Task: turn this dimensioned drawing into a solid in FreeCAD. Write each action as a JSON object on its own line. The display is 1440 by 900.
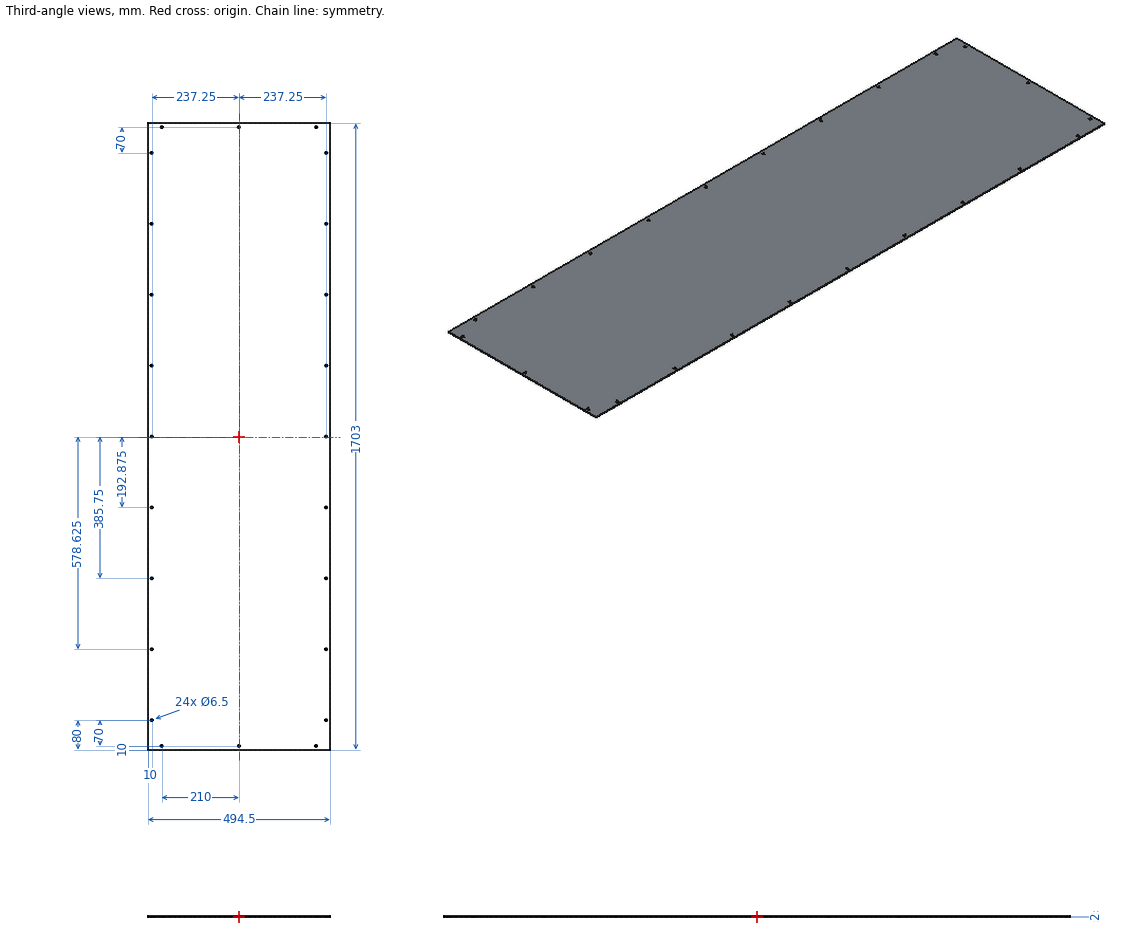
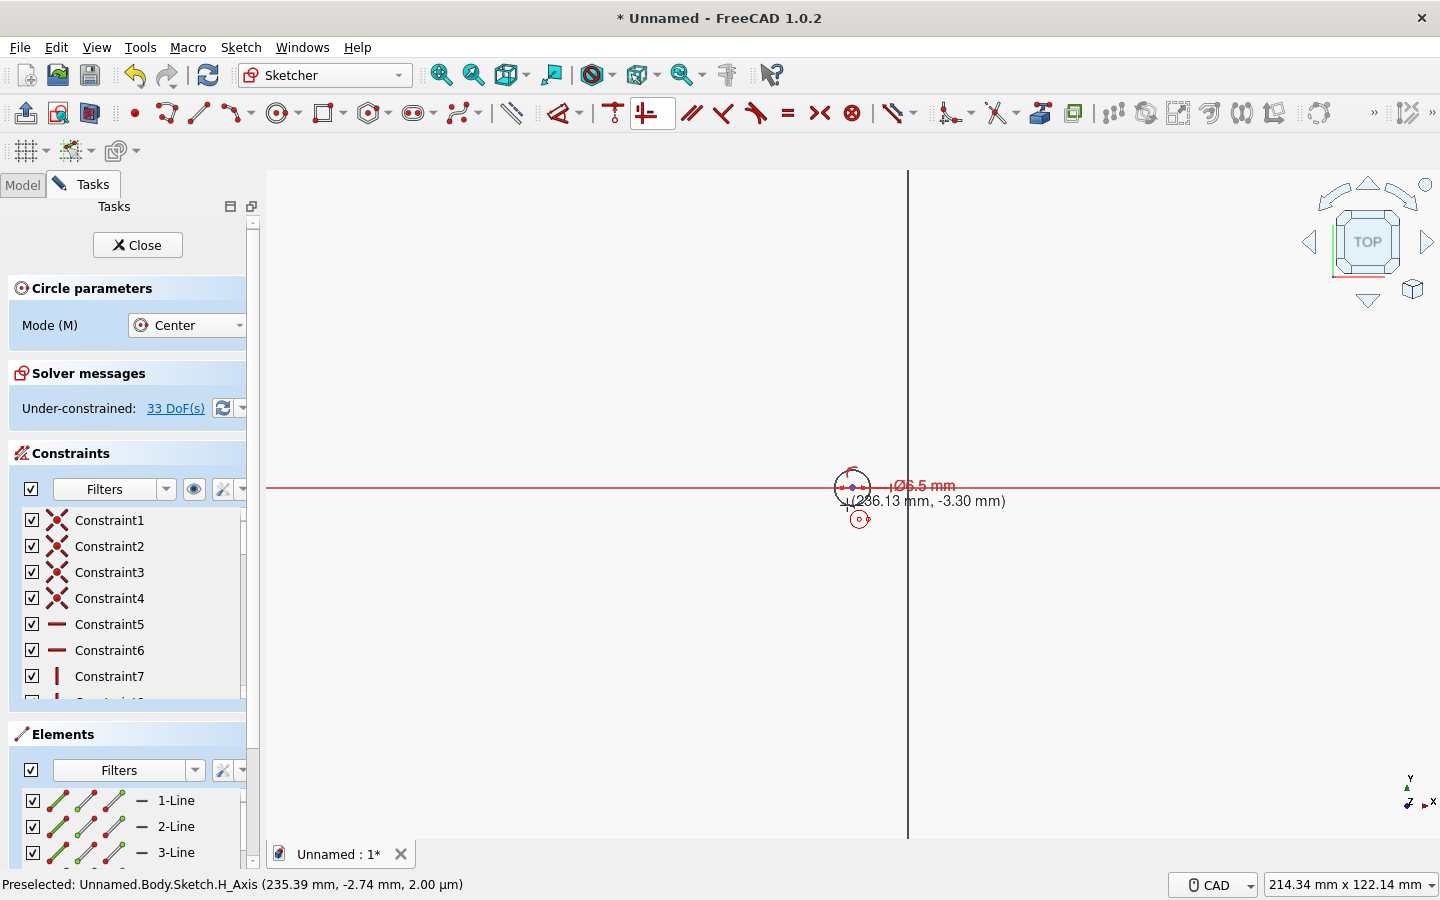
{"action": "scroll", "coordinate": [849, 505], "scroll_direction": "down", "scroll_amount": 15}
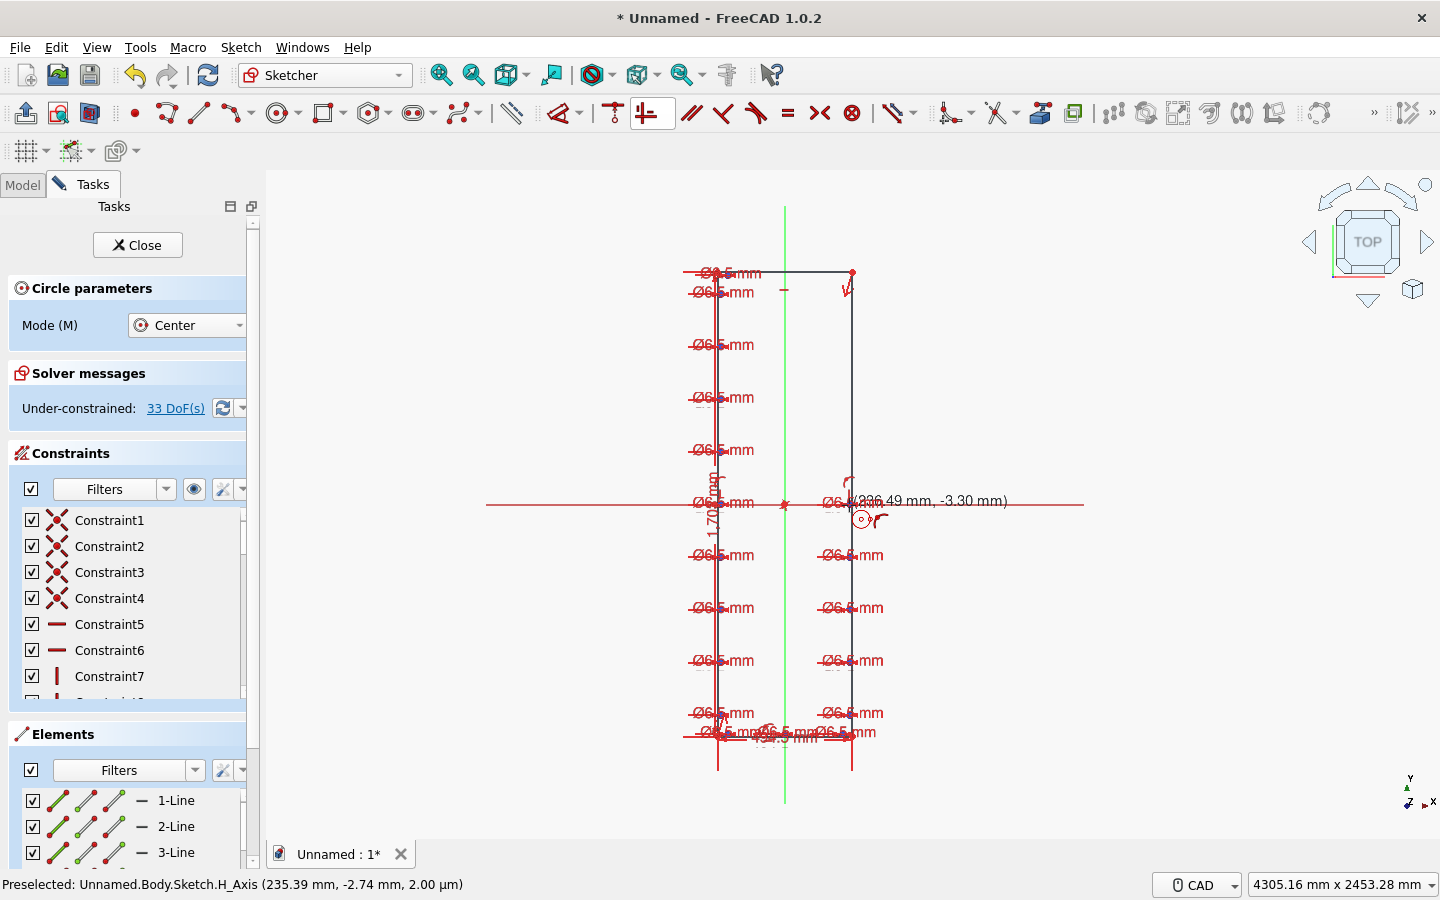
{"action": "scroll", "coordinate": [850, 452], "scroll_direction": "up", "scroll_amount": 17}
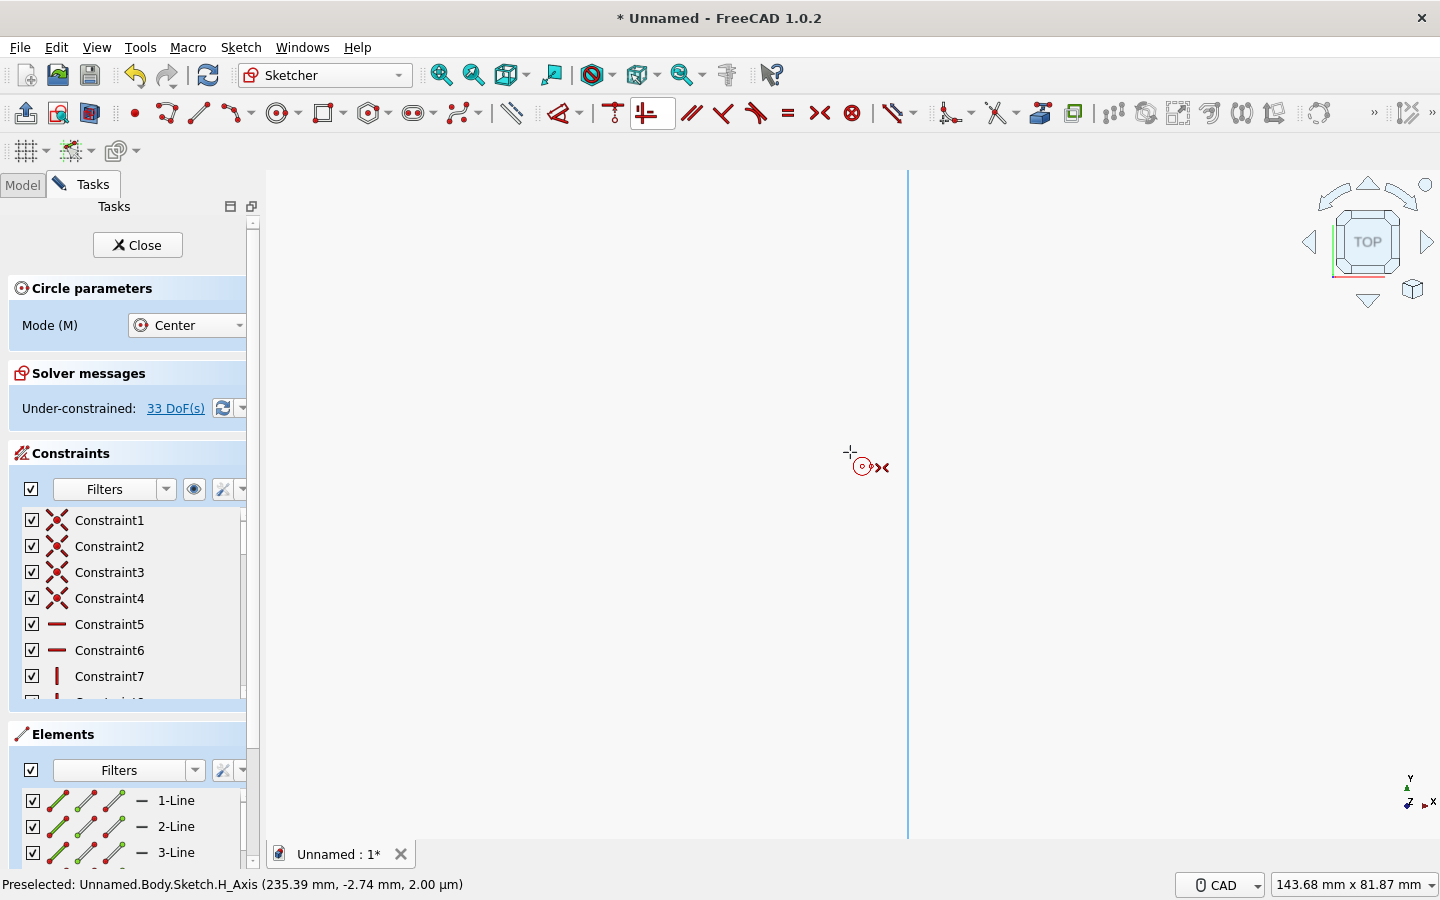
{"action": "scroll", "coordinate": [850, 452], "scroll_direction": "down", "scroll_amount": 17}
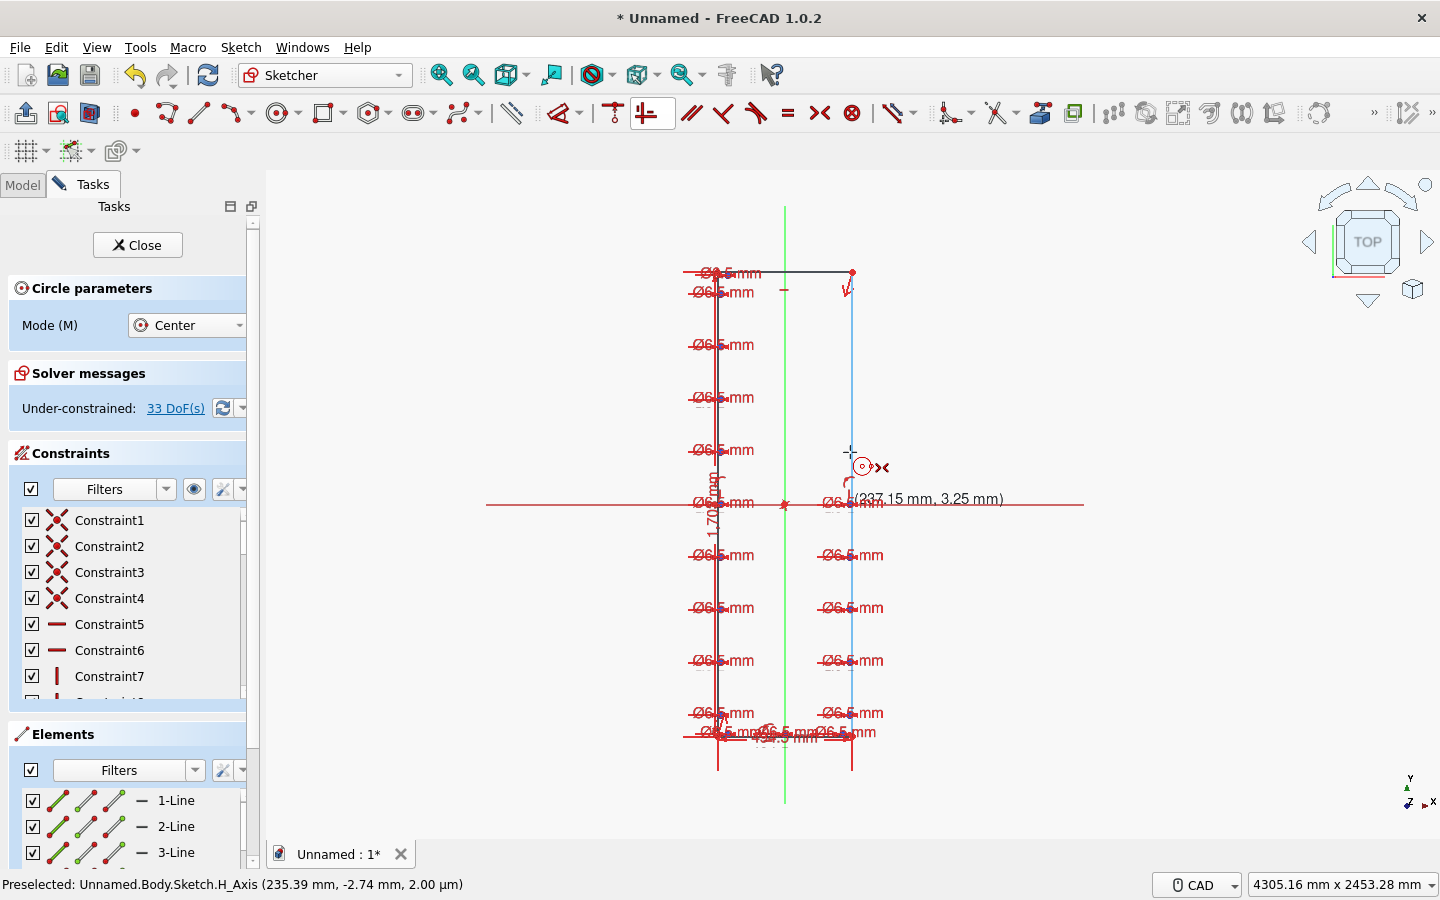
{"action": "scroll", "coordinate": [850, 452], "scroll_direction": "up", "scroll_amount": 9}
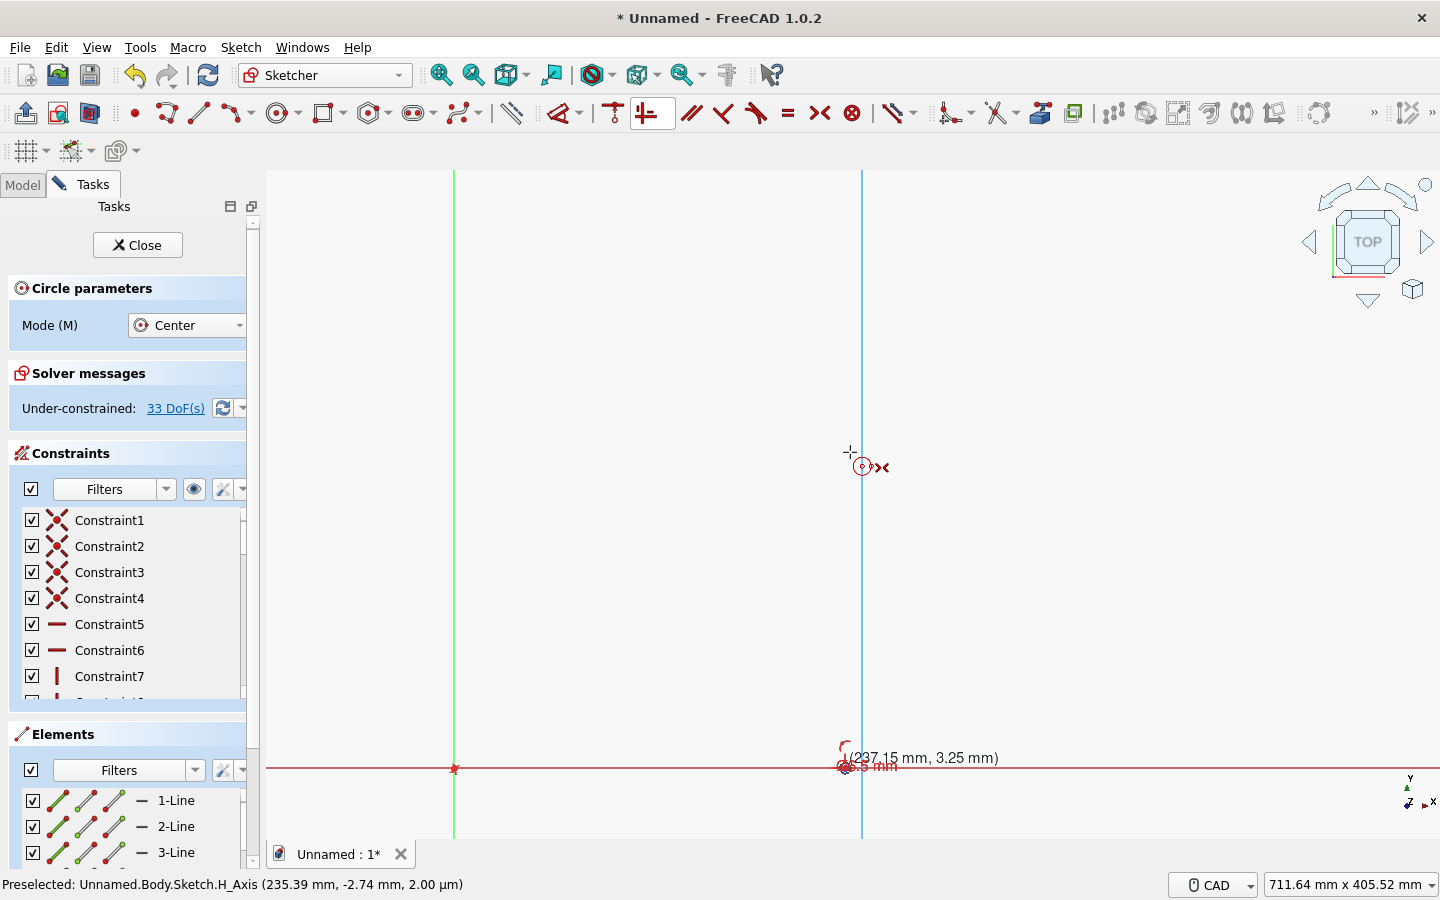
{"action": "left_click", "coordinate": [846, 450]}
{"action": "mouse_move", "coordinate": [842, 446]}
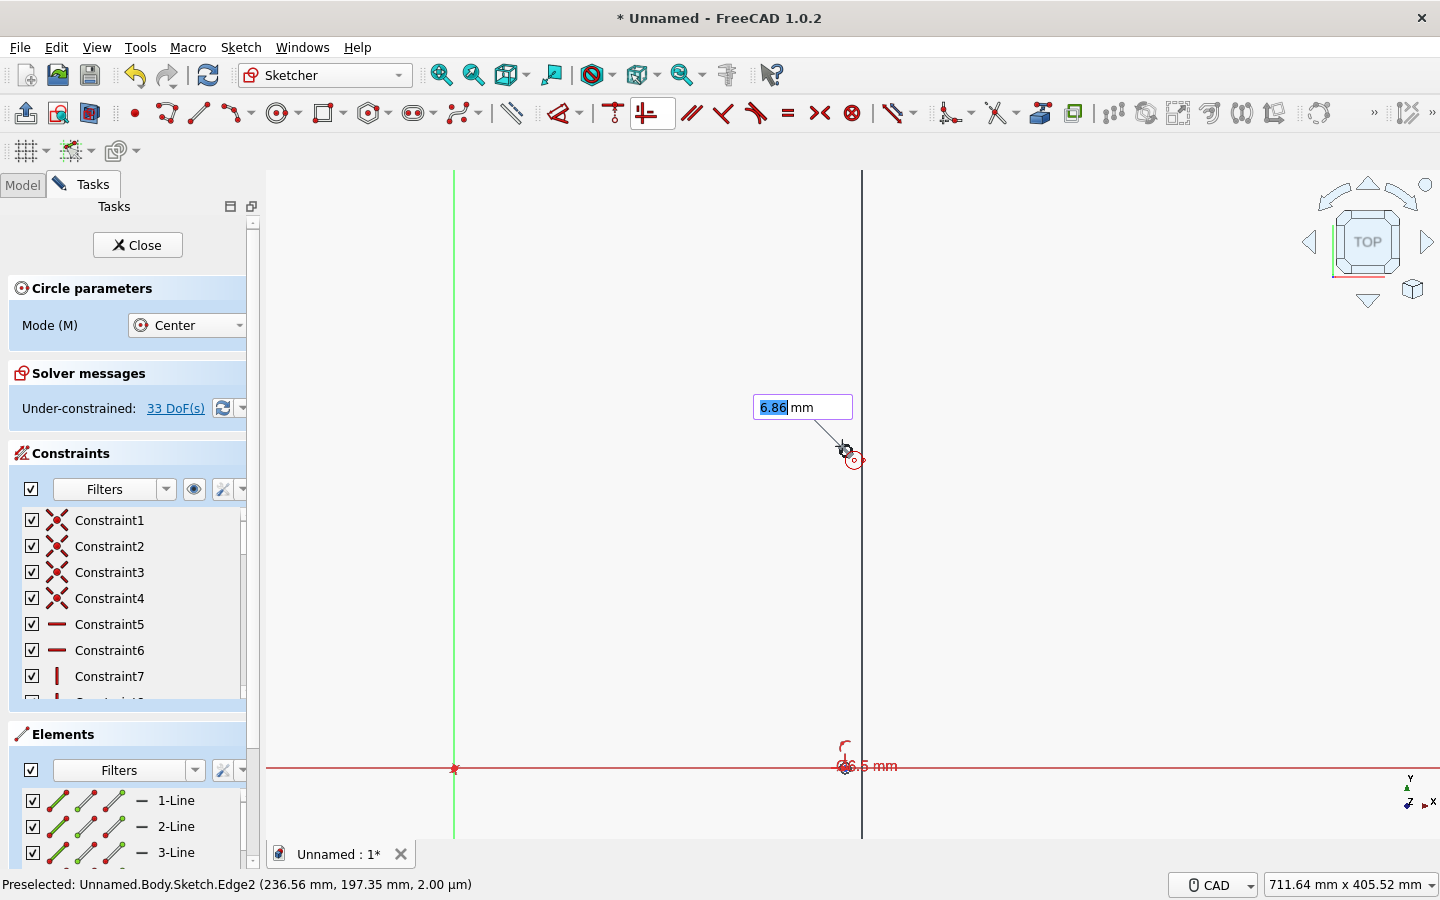
{"action": "type", "text": "6.5"}
{"action": "key", "text": "Return"}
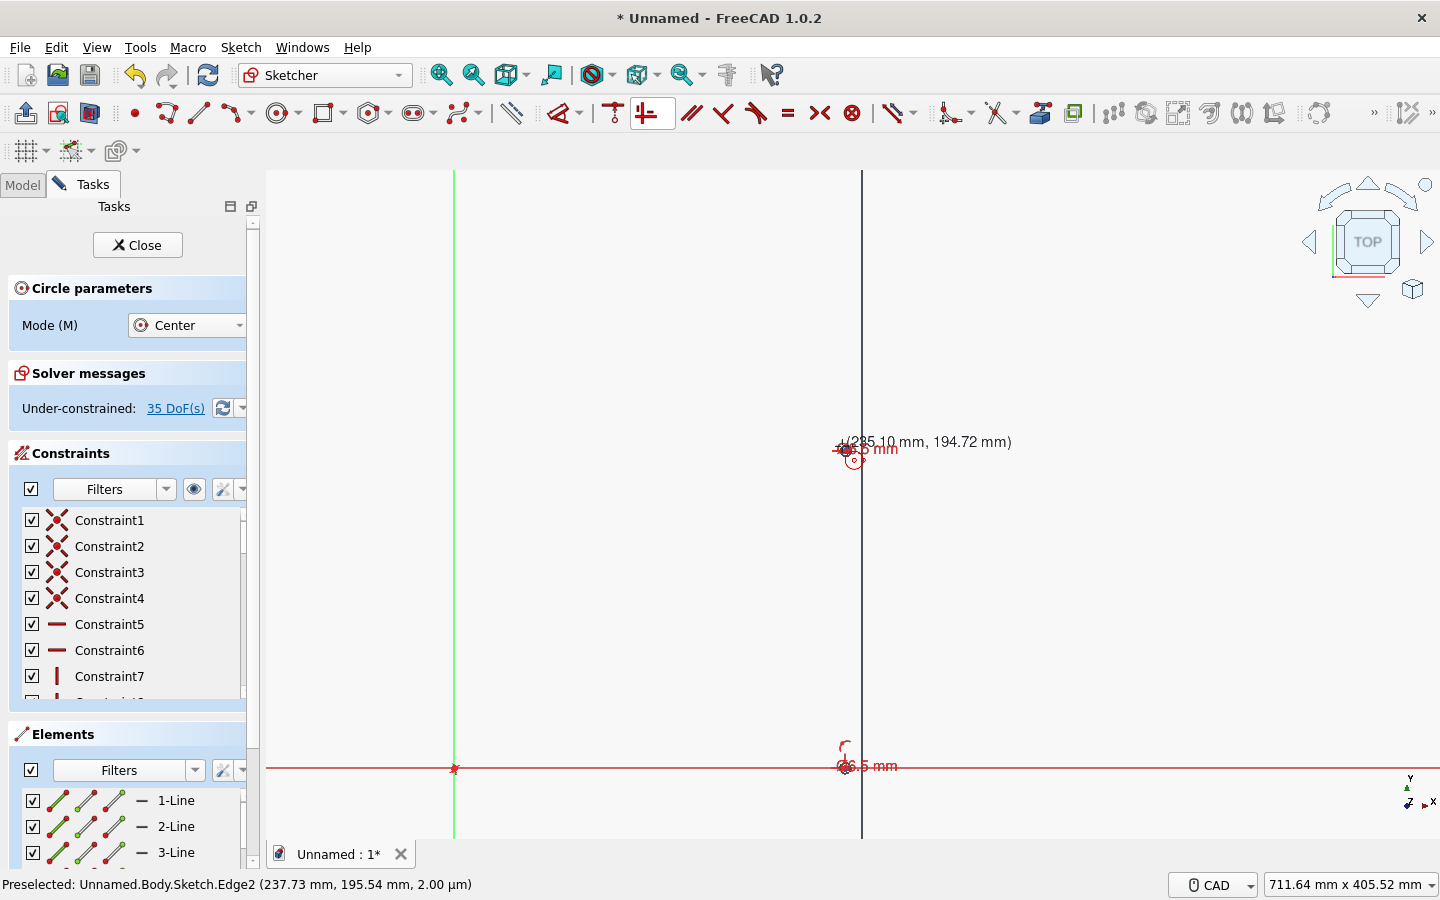
{"action": "scroll", "coordinate": [850, 452], "scroll_direction": "down", "scroll_amount": 9}